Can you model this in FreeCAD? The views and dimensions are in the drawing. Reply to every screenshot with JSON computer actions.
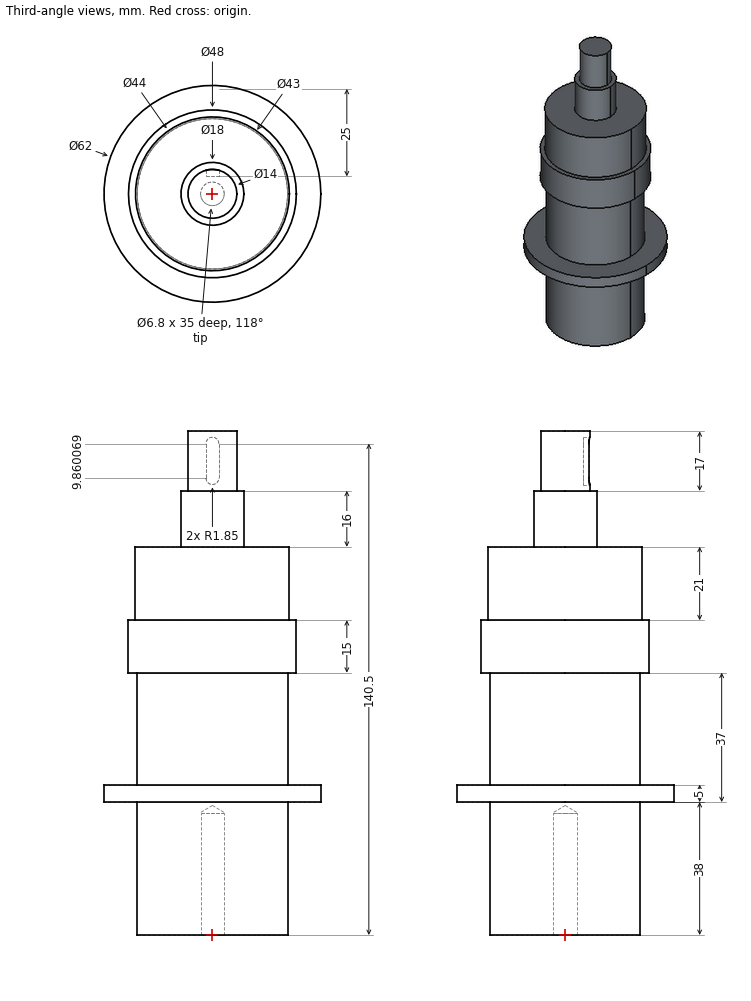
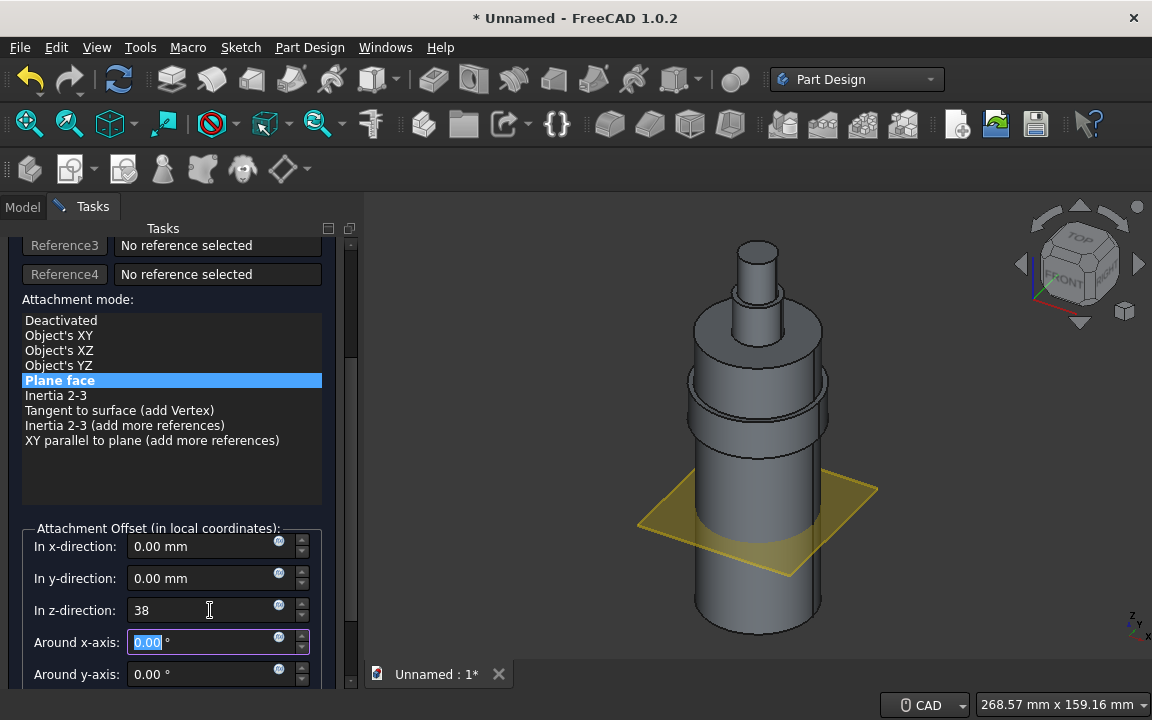
{"action": "scroll", "coordinate": [351, 463], "scroll_direction": "up", "scroll_amount": 4}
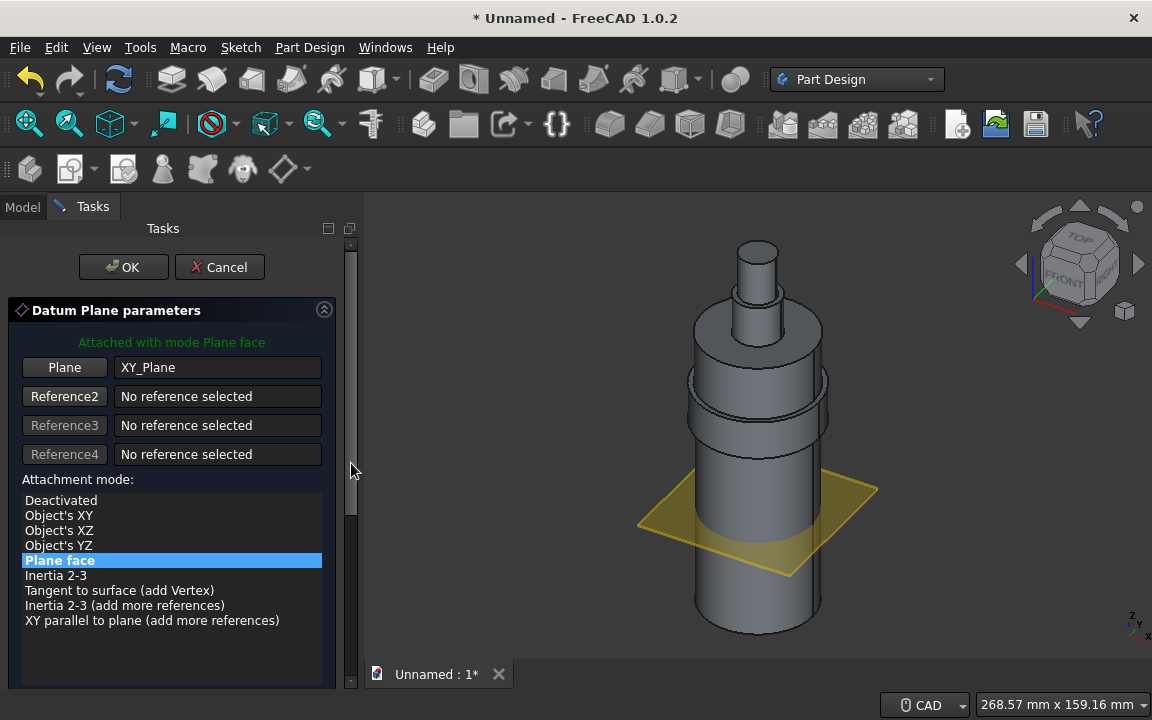
{"action": "left_click", "coordinate": [124, 267]}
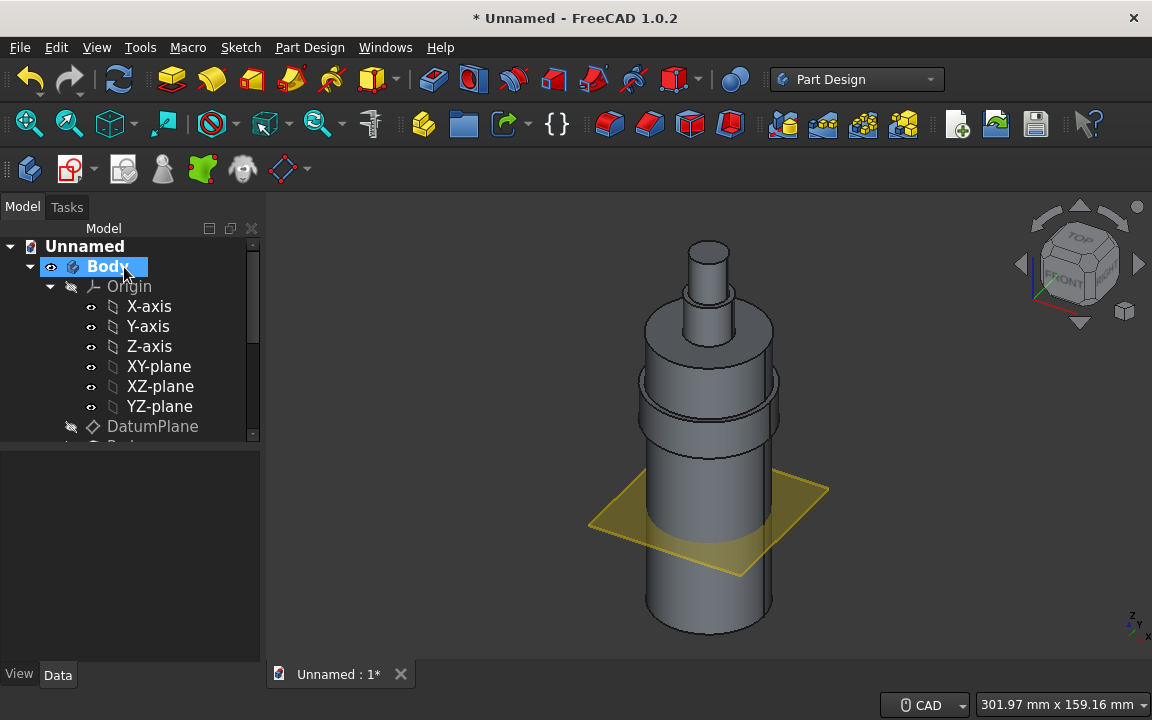
{"action": "scroll", "coordinate": [100, 342], "scroll_direction": "down", "scroll_amount": 3}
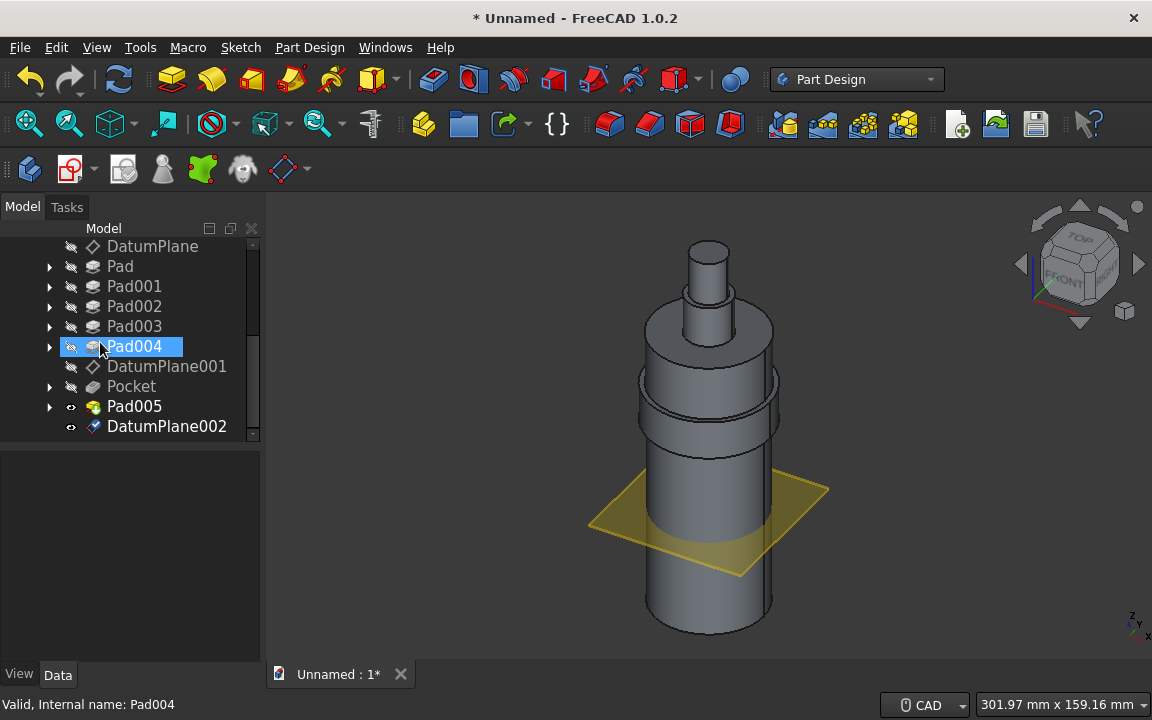
{"action": "left_click", "coordinate": [116, 427]}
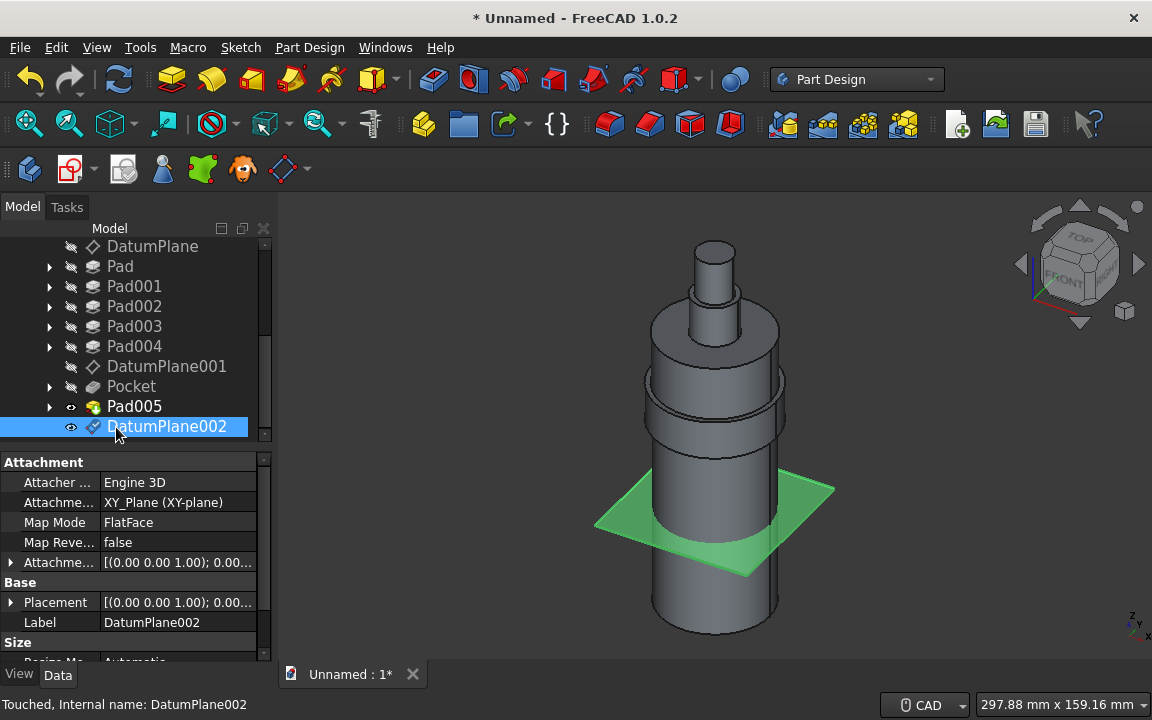
{"action": "left_click", "coordinate": [70, 170]}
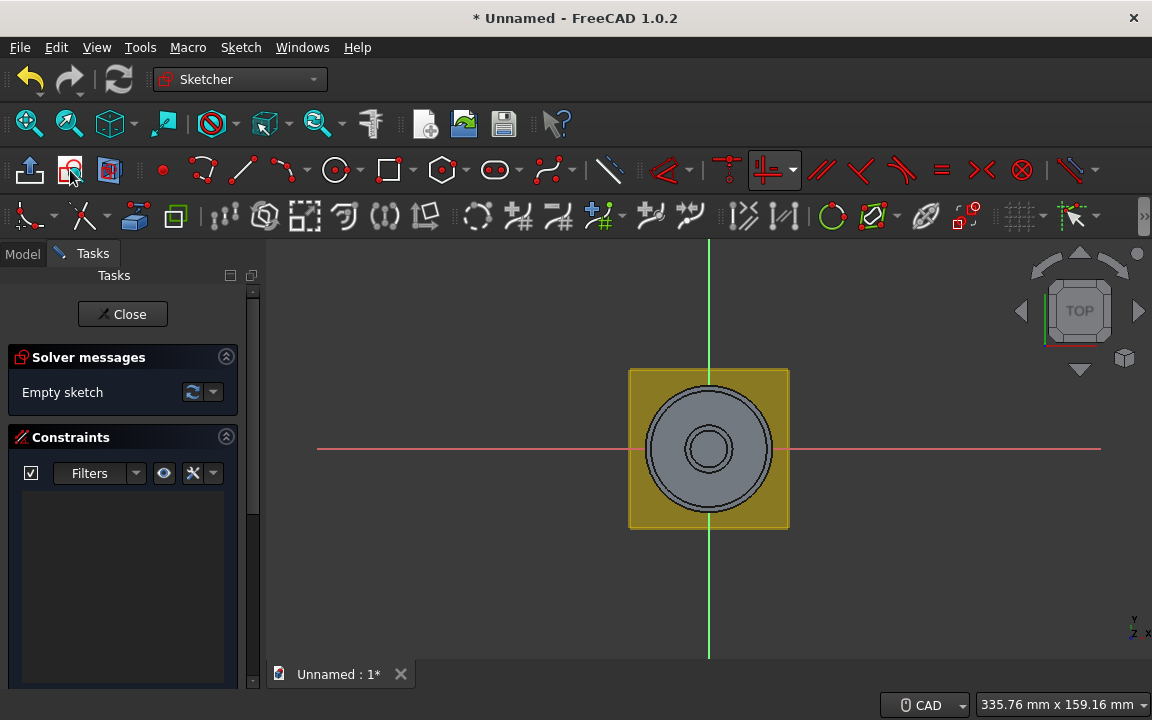
{"action": "left_click", "coordinate": [110, 170]}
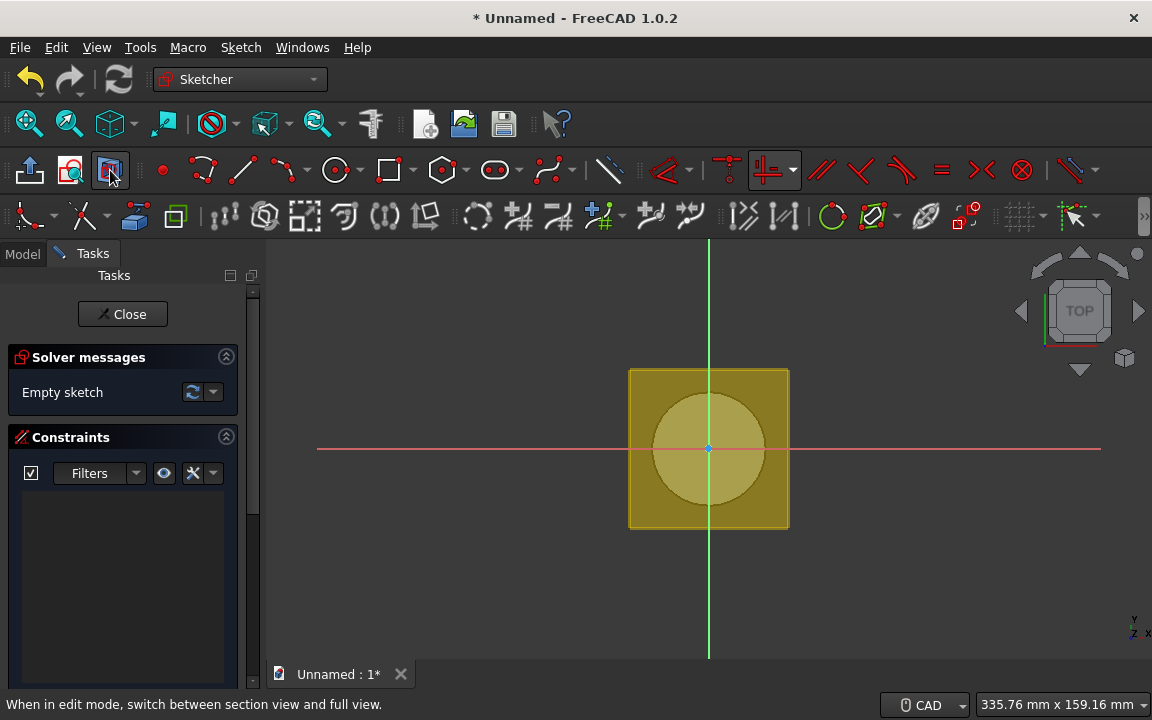
{"action": "scroll", "coordinate": [848, 449], "scroll_direction": "up", "scroll_amount": 2}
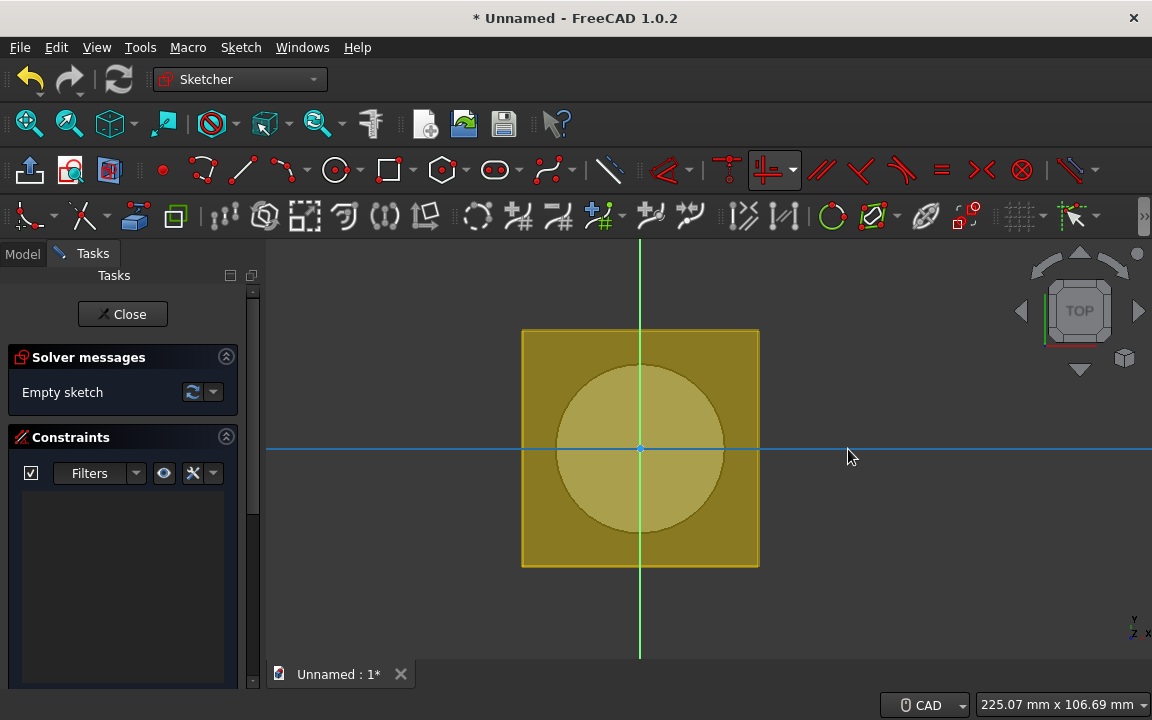
{"action": "left_click", "coordinate": [336, 170]}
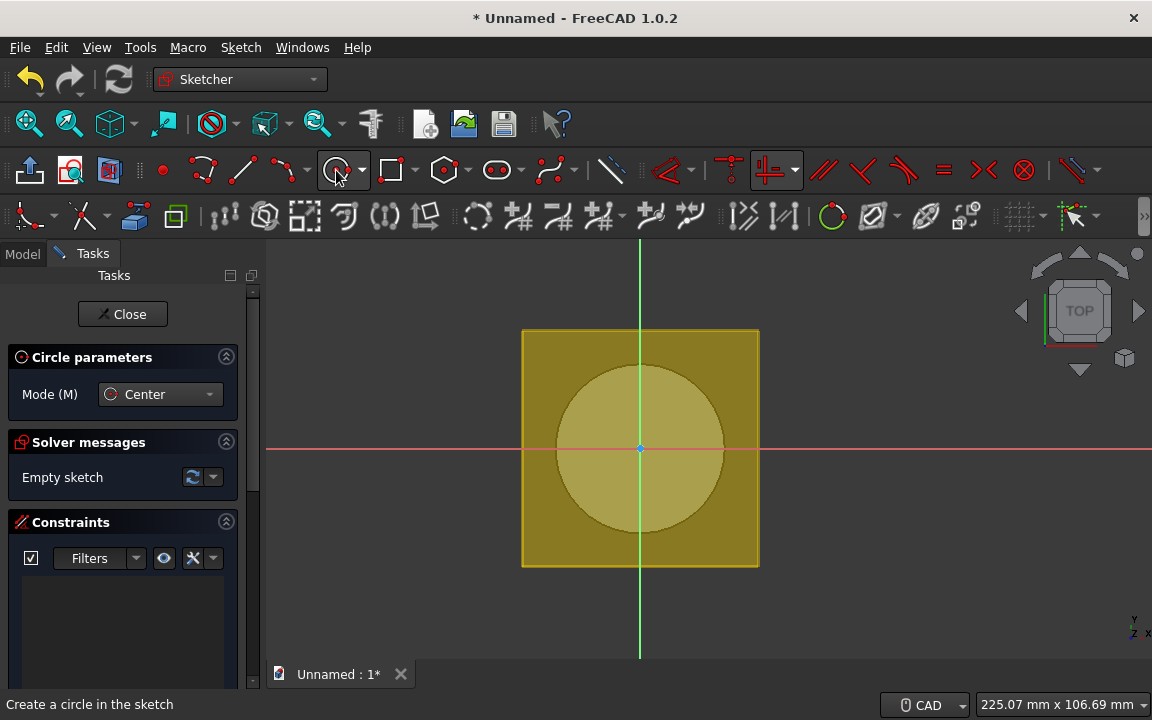
{"action": "left_click", "coordinate": [640, 449]}
{"action": "left_click", "coordinate": [726, 362]}
{"action": "key", "text": "Escape"}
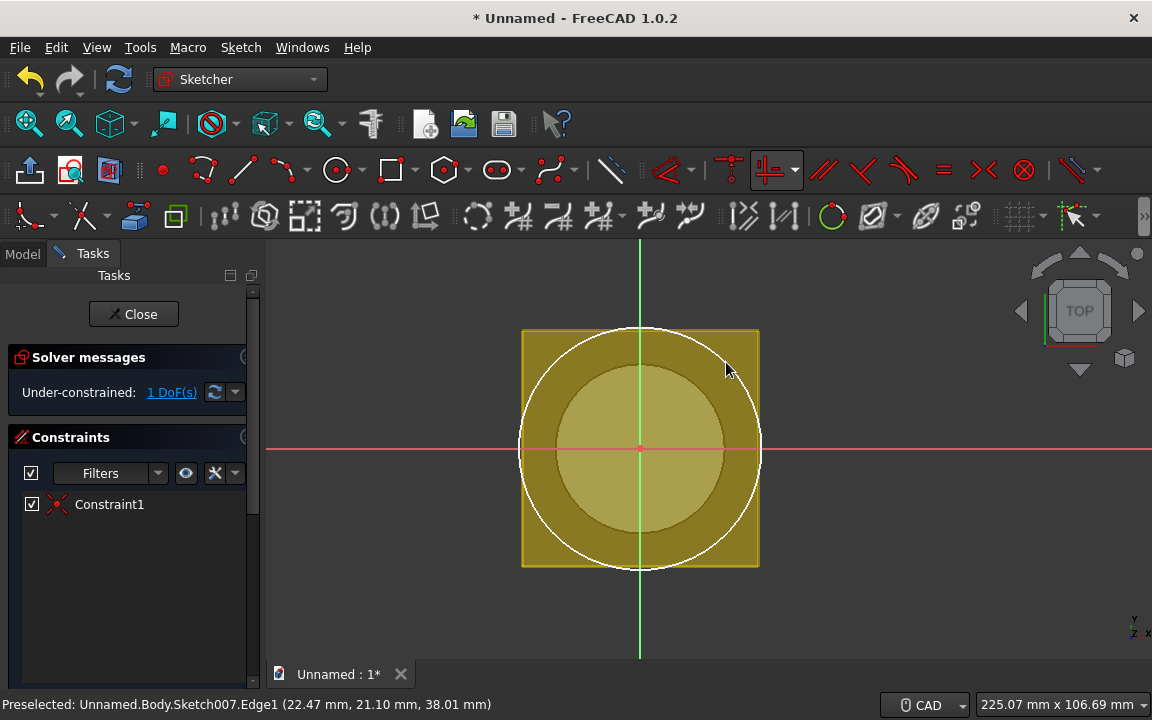
{"action": "left_click", "coordinate": [666, 170]}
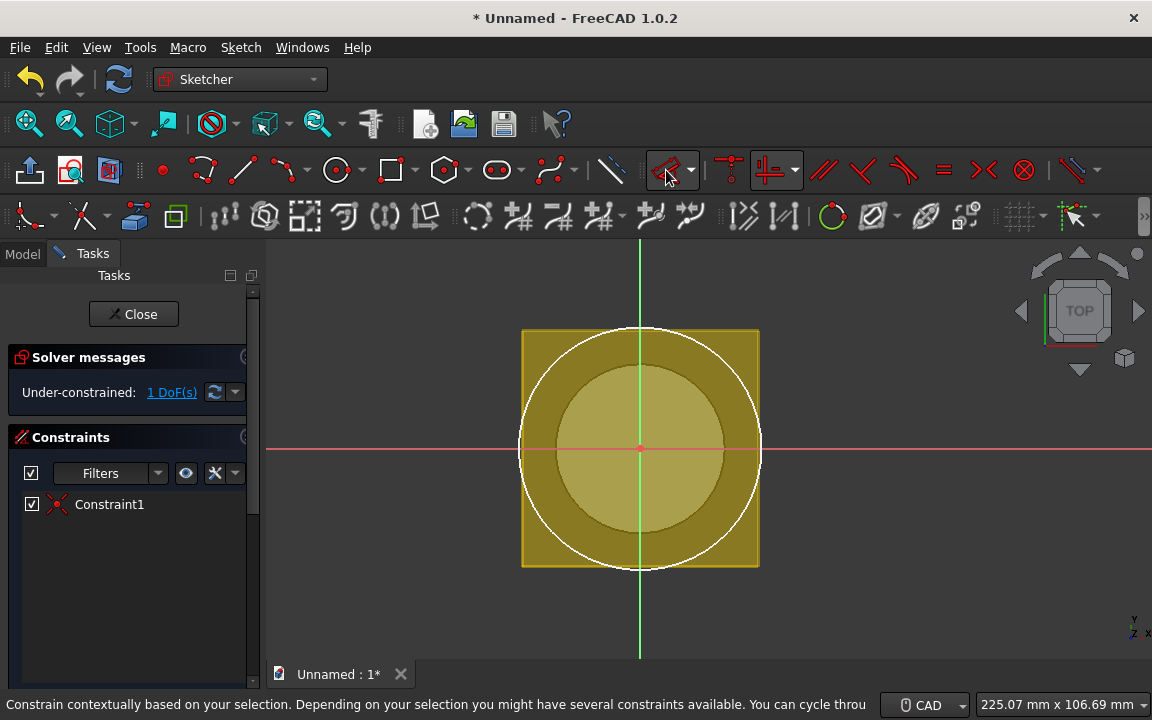
{"action": "left_click", "coordinate": [726, 363]}
{"action": "left_click", "coordinate": [749, 340]}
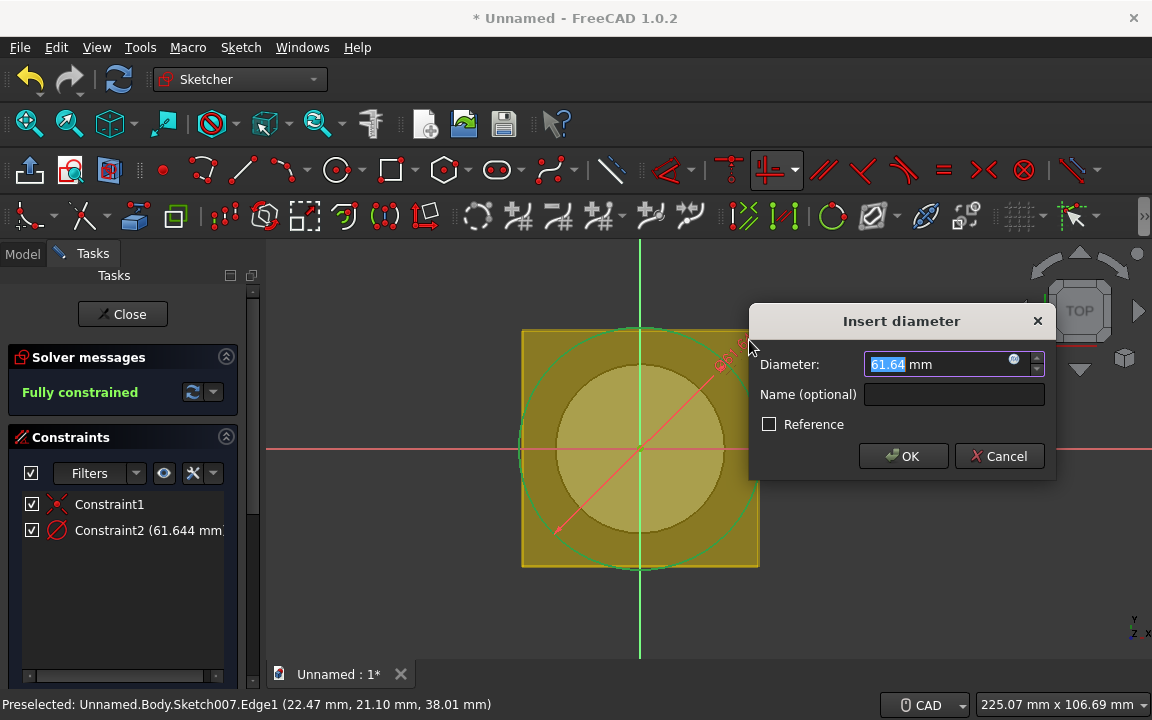
{"action": "type", "text": "62"}
{"action": "key", "text": "Return"}
{"action": "key", "text": "Escape"}